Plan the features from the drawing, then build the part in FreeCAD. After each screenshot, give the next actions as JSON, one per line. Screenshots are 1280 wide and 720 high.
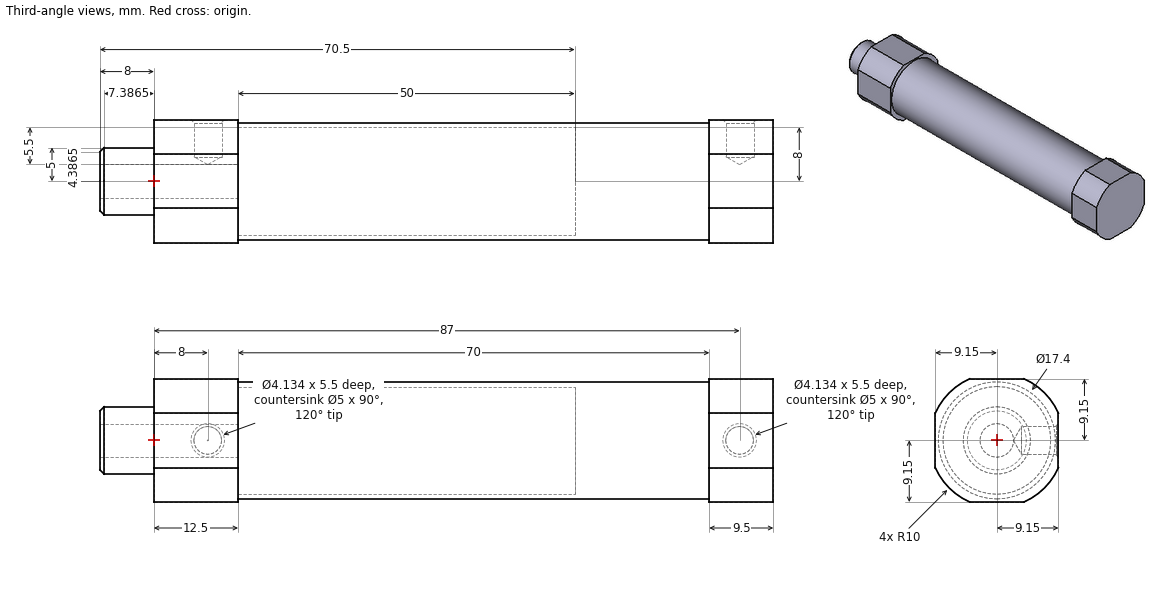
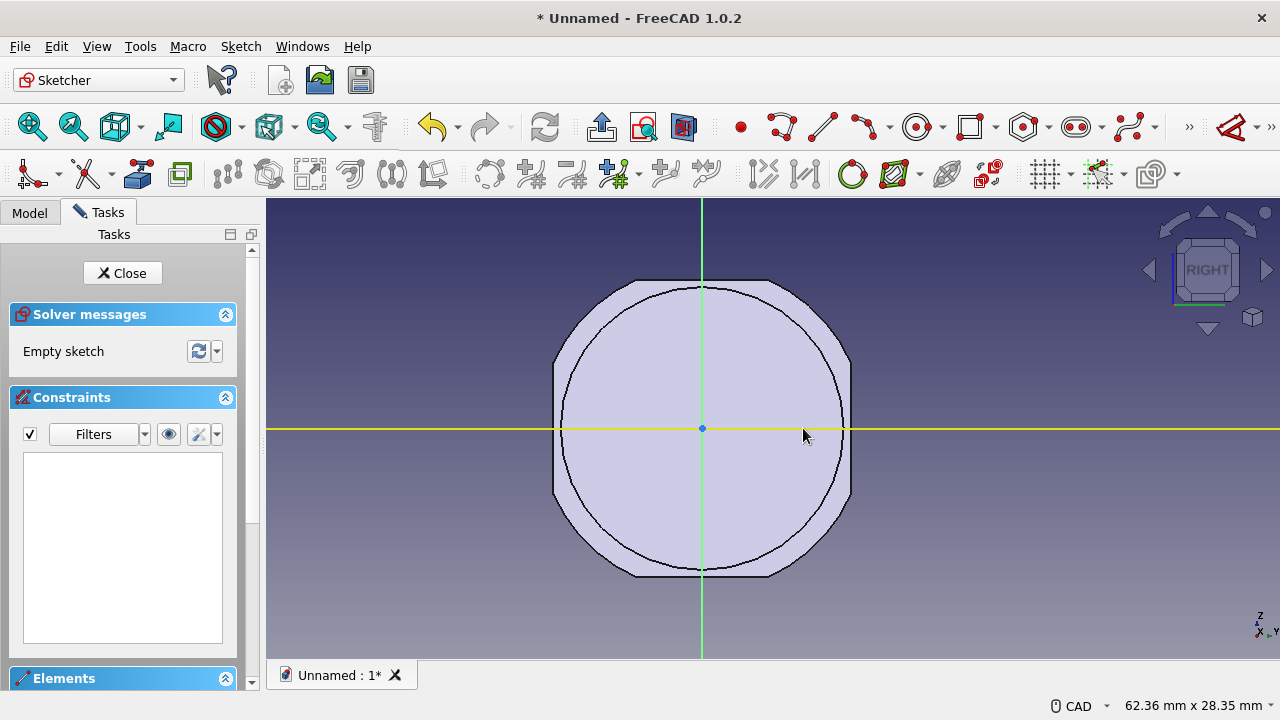
{"action": "left_click", "coordinate": [823, 128]}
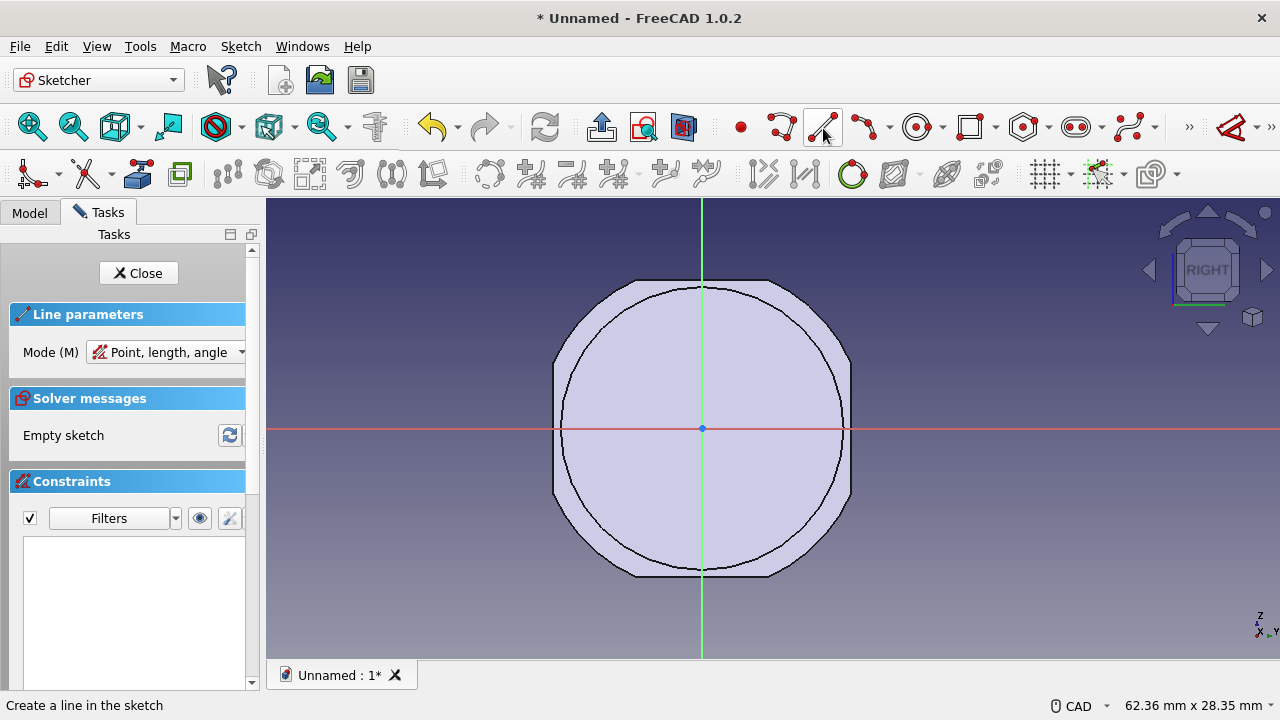
{"action": "left_click", "coordinate": [553, 363]}
{"action": "left_click", "coordinate": [553, 494]}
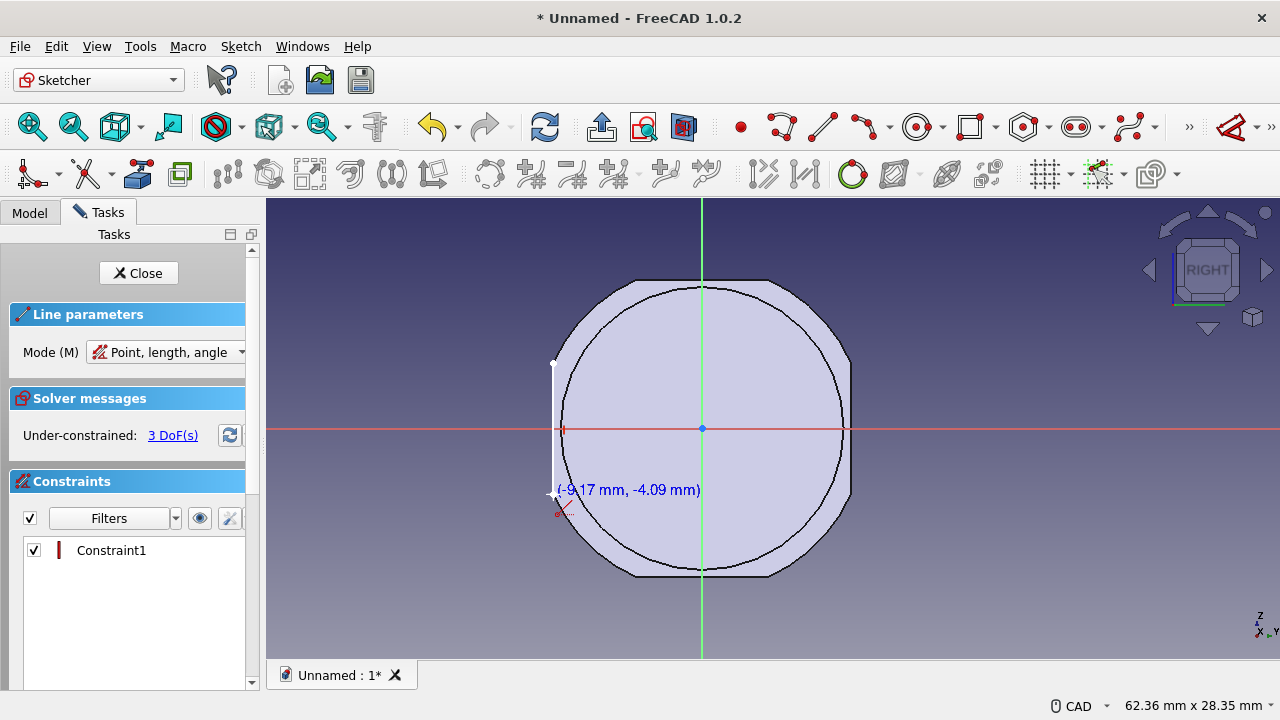
{"action": "left_click", "coordinate": [637, 577]}
{"action": "left_click", "coordinate": [768, 577]}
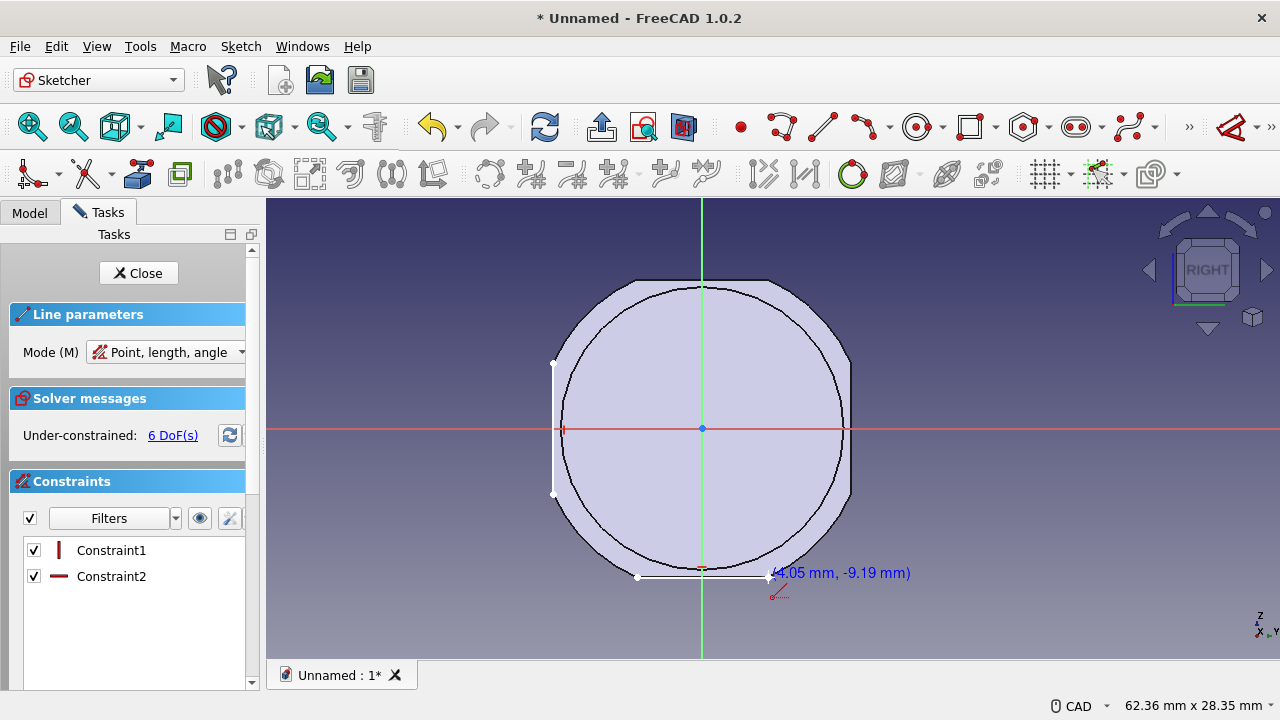
{"action": "left_click", "coordinate": [851, 494]}
{"action": "left_click", "coordinate": [851, 363]}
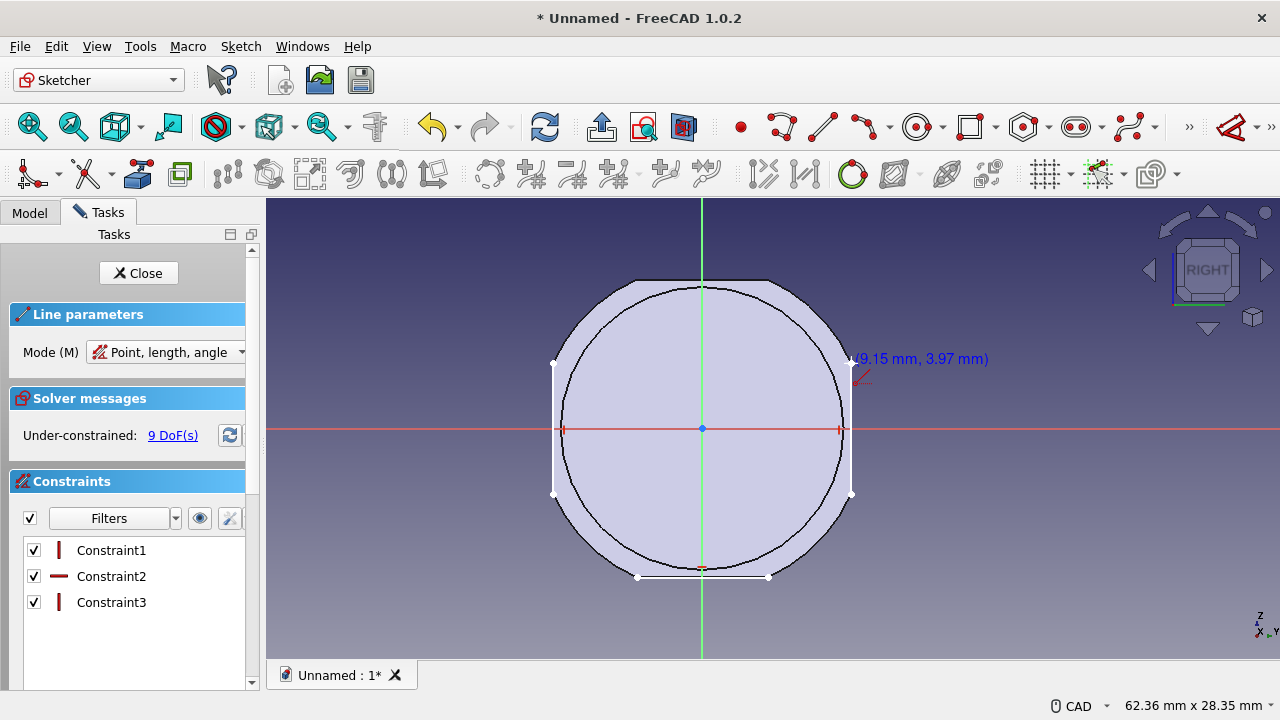
{"action": "left_click", "coordinate": [768, 280]}
{"action": "left_click", "coordinate": [637, 280]}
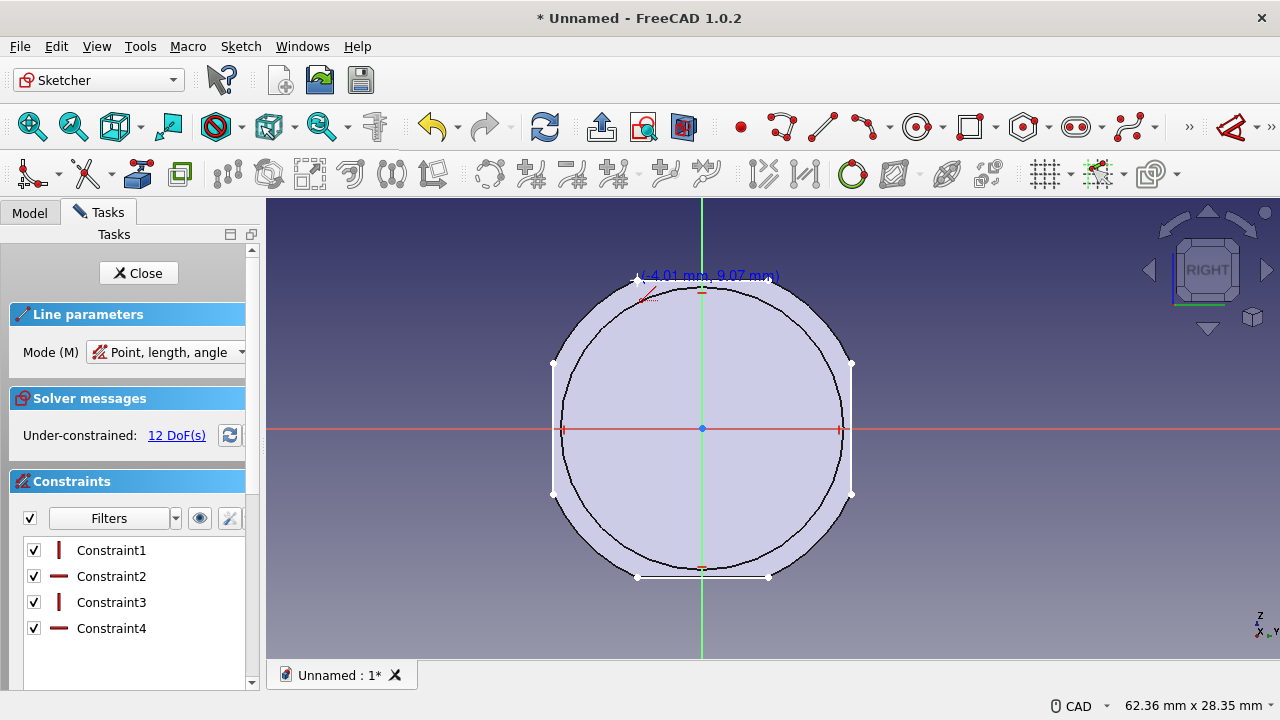
{"action": "left_click", "coordinate": [864, 128]}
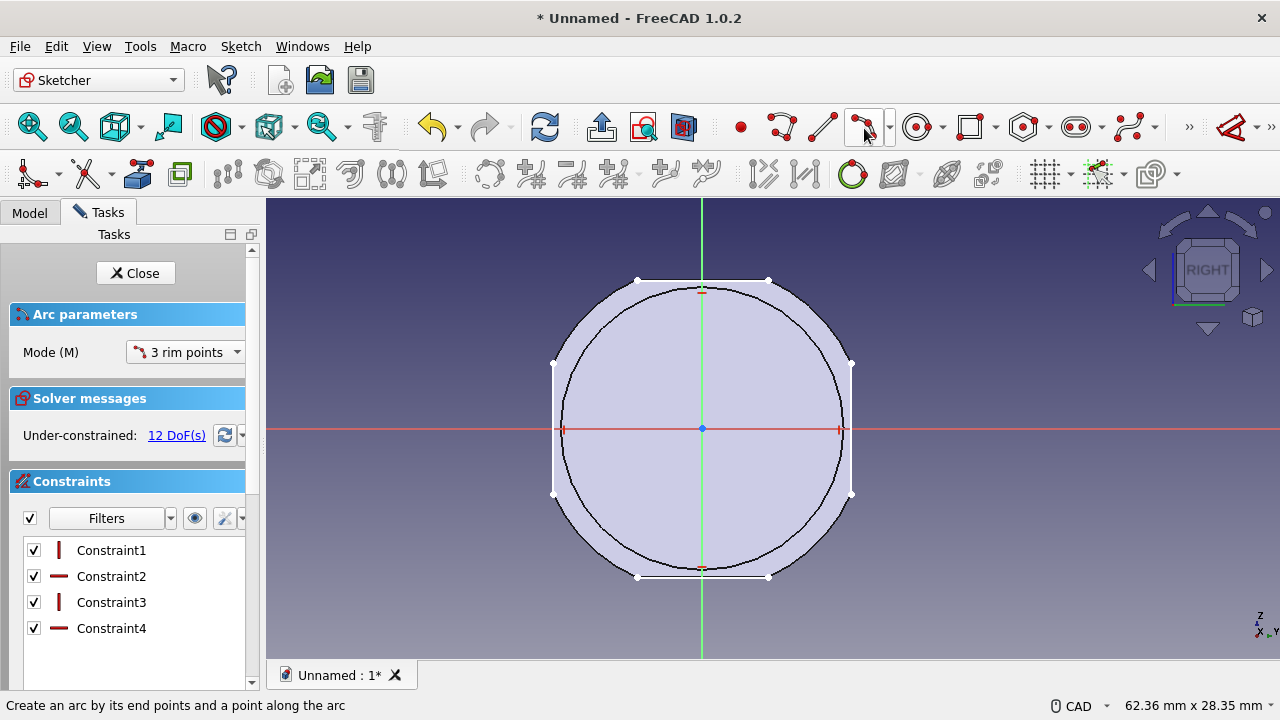
{"action": "left_click", "coordinate": [553, 495]}
{"action": "left_click", "coordinate": [637, 578]}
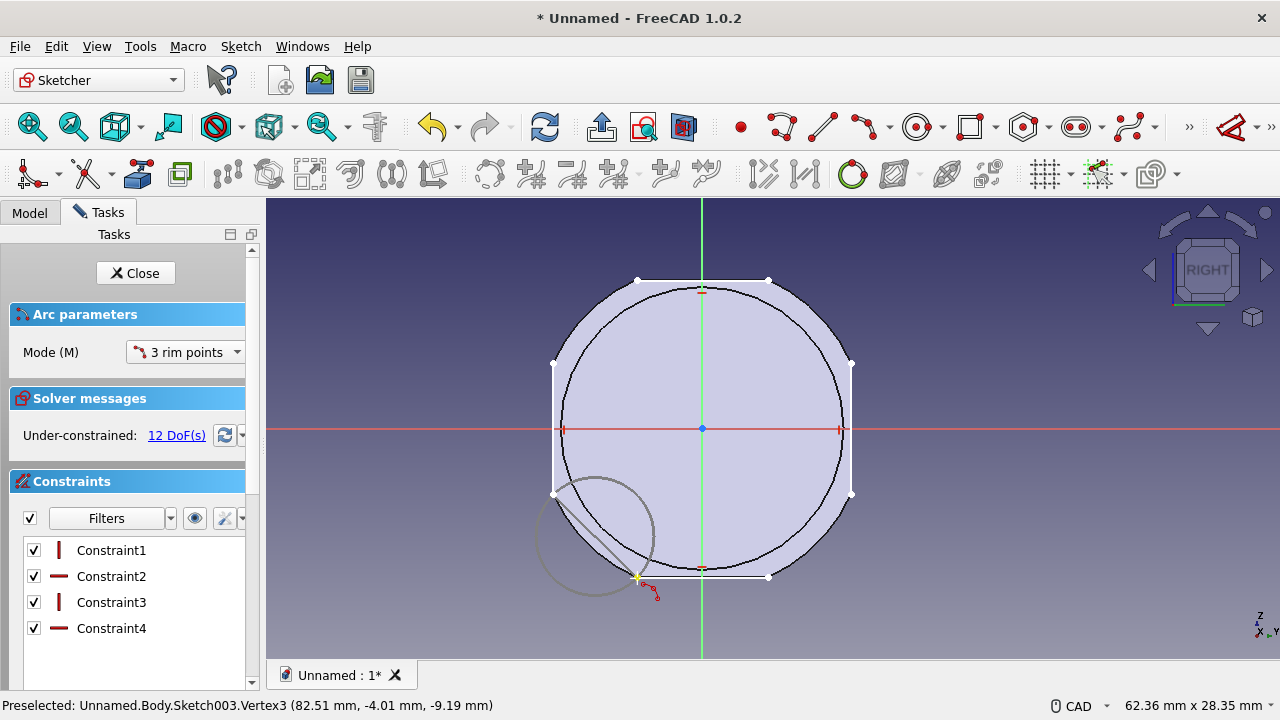
{"action": "scroll", "coordinate": [587, 543], "scroll_direction": "up", "scroll_amount": 2}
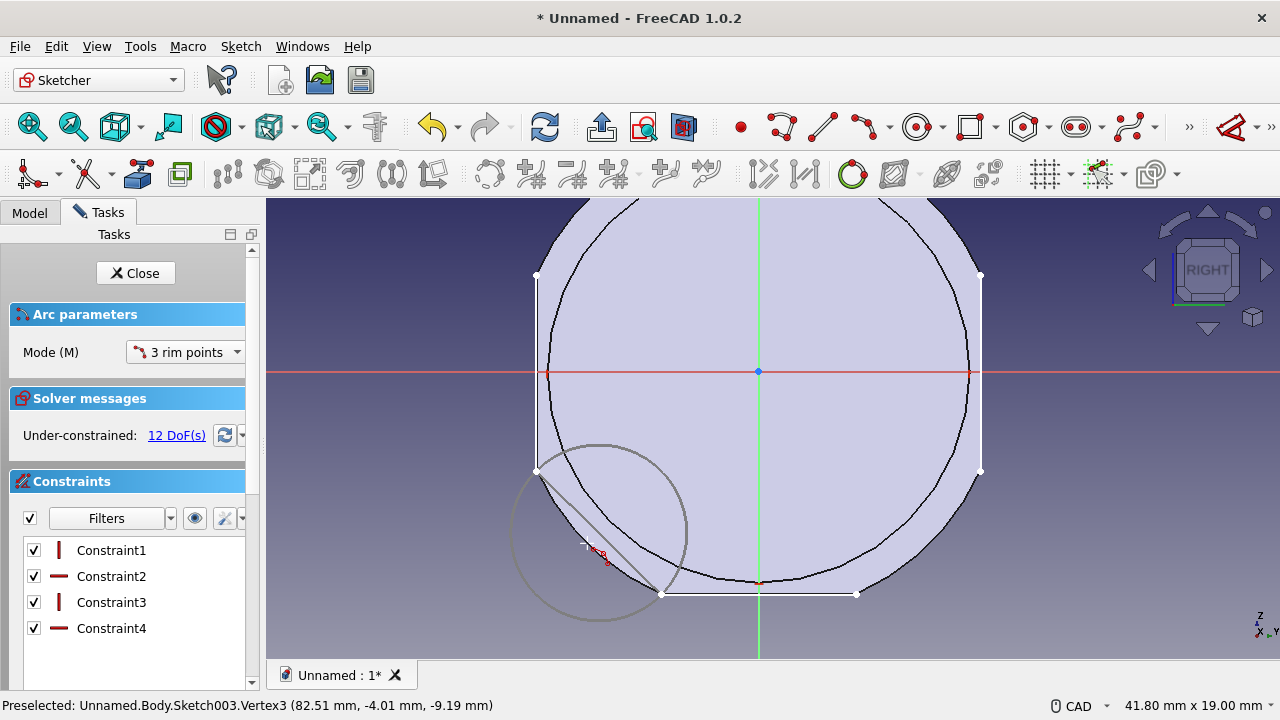
{"action": "left_click", "coordinate": [587, 543]}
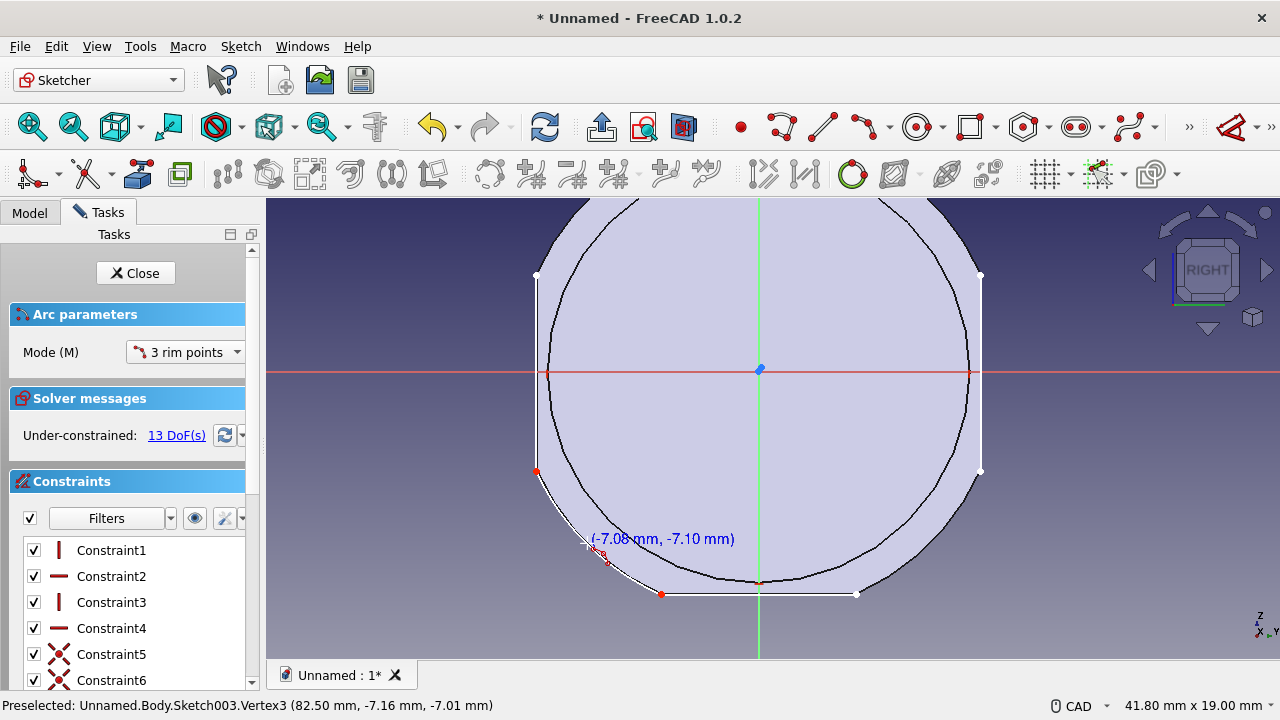
{"action": "left_click", "coordinate": [857, 595]}
{"action": "left_click", "coordinate": [981, 471]}
{"action": "left_click", "coordinate": [930, 543]}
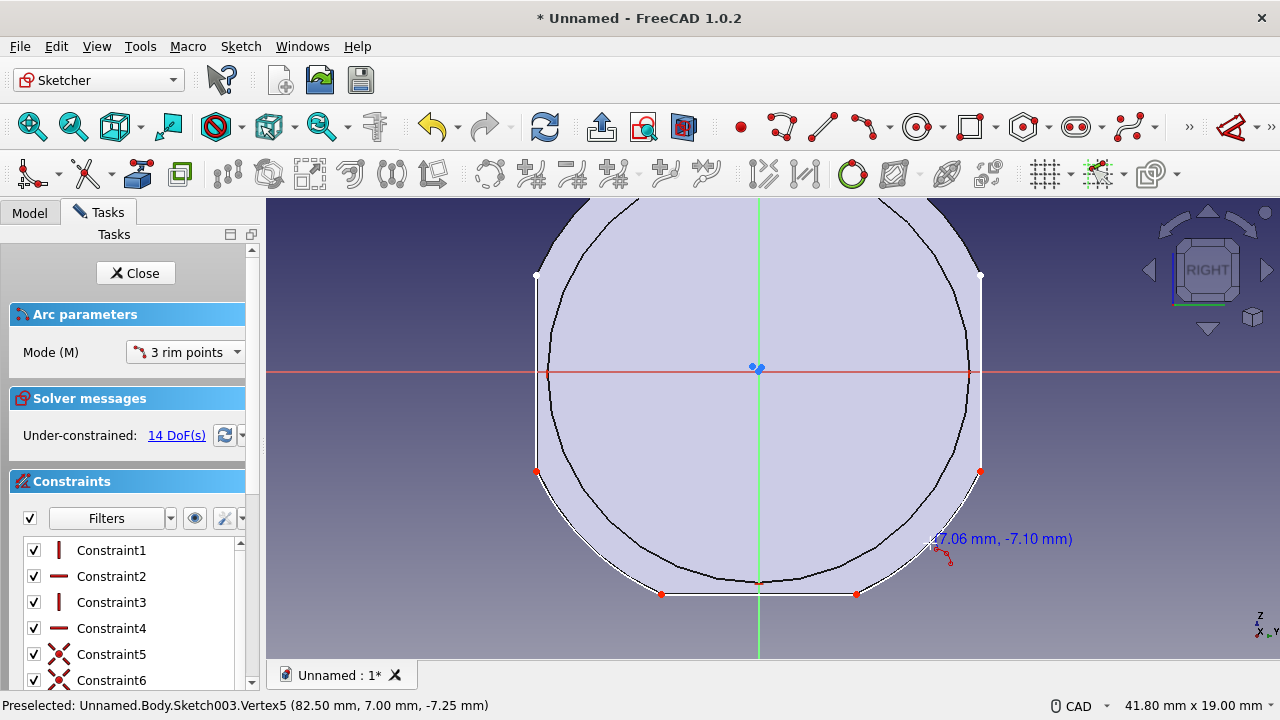
{"action": "left_click", "coordinate": [981, 276]}